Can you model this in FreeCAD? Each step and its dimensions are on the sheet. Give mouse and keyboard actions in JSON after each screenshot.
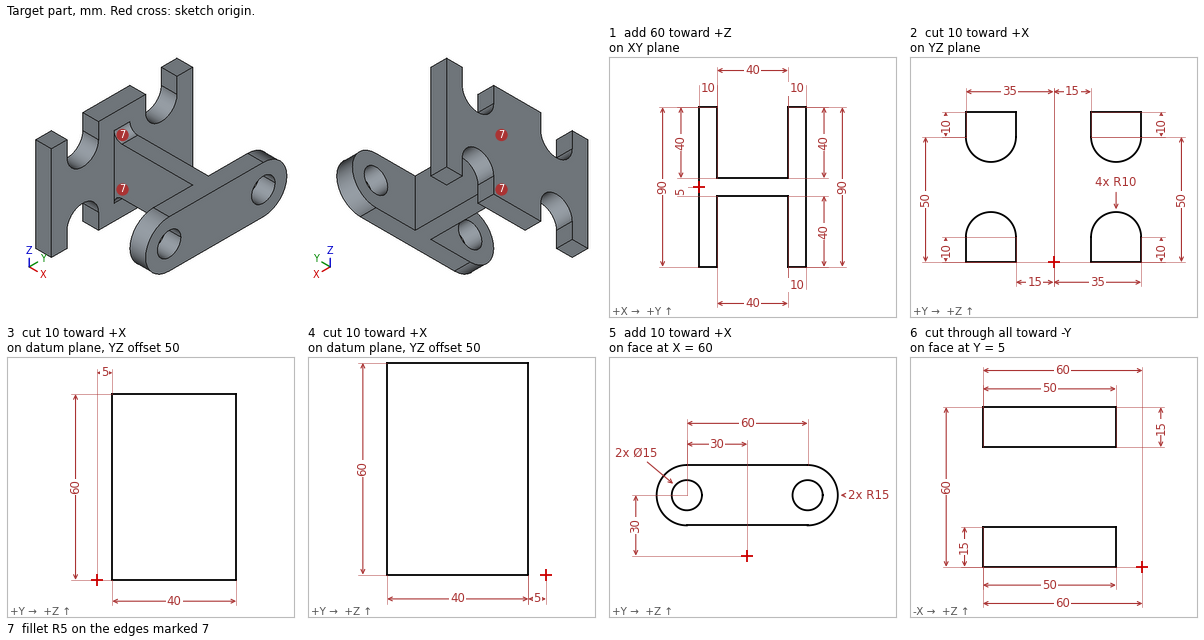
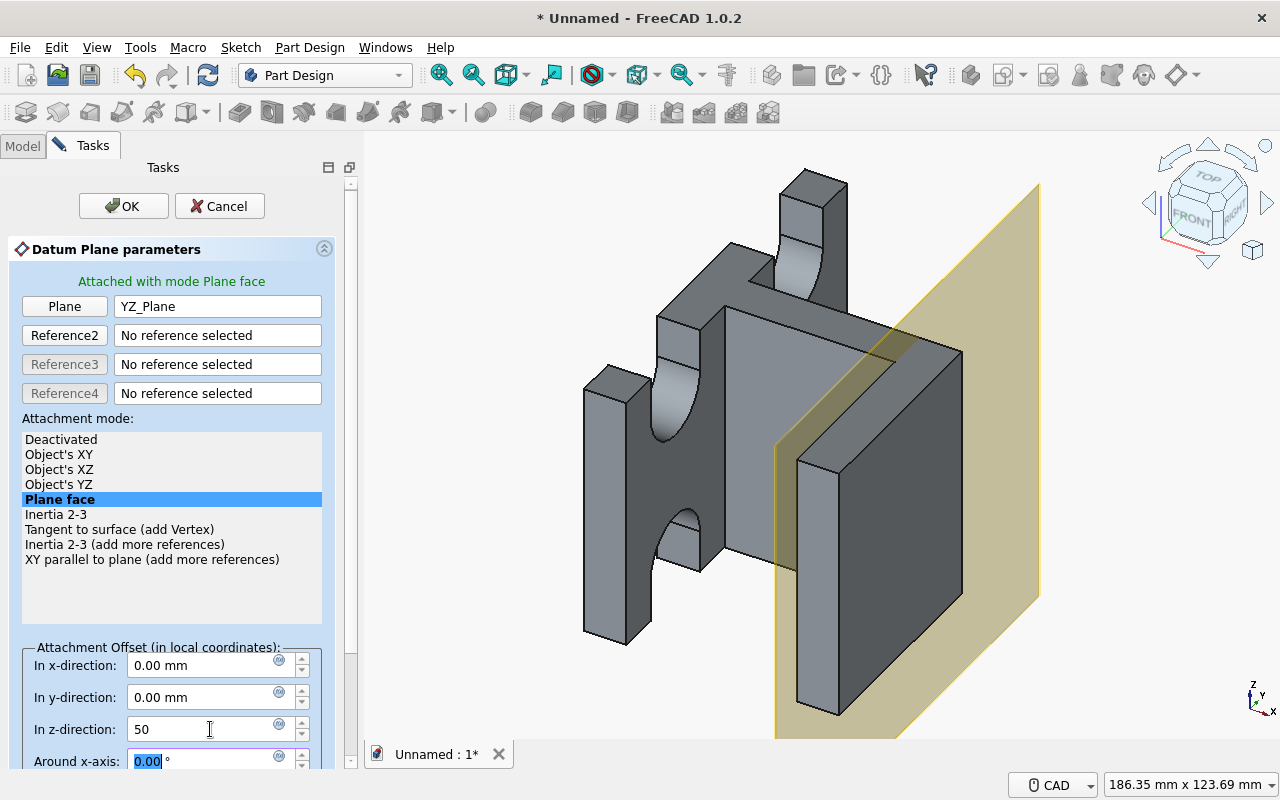
{"action": "left_click", "coordinate": [124, 206]}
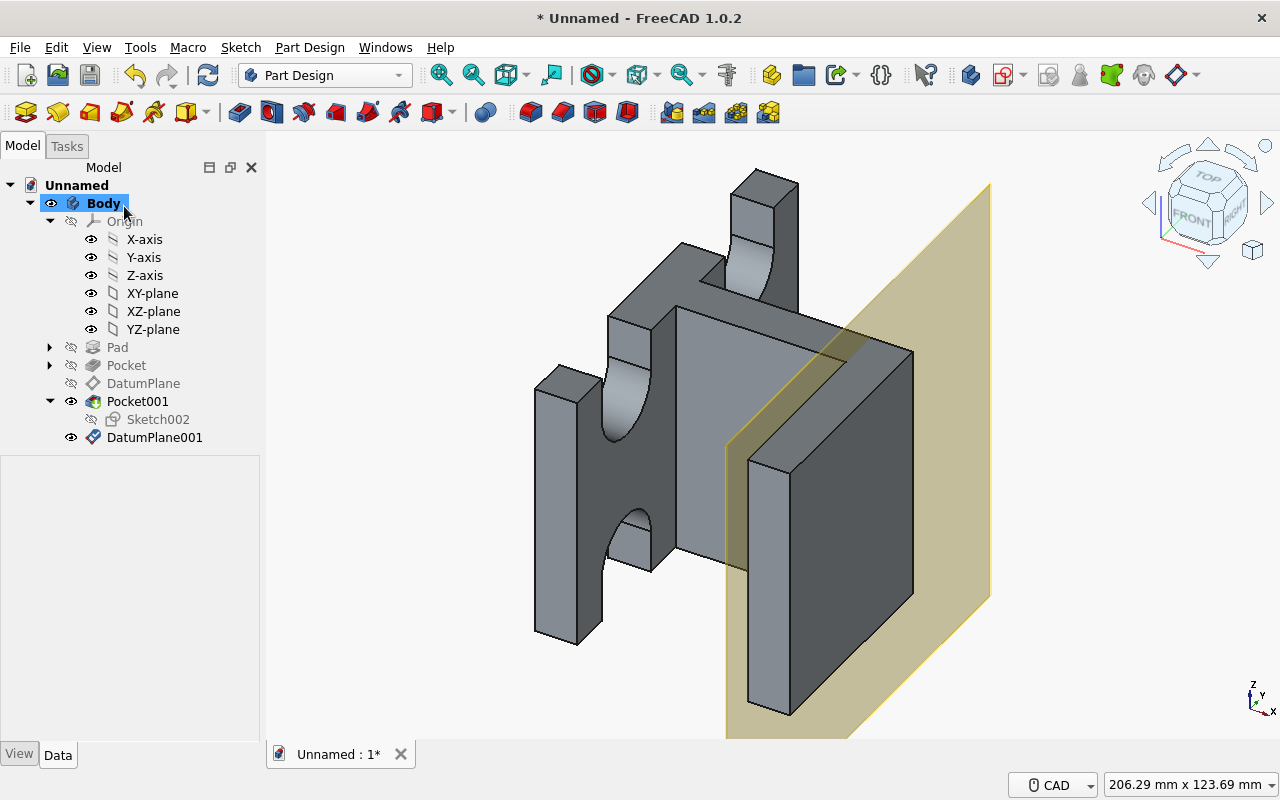
{"action": "left_click", "coordinate": [116, 437]}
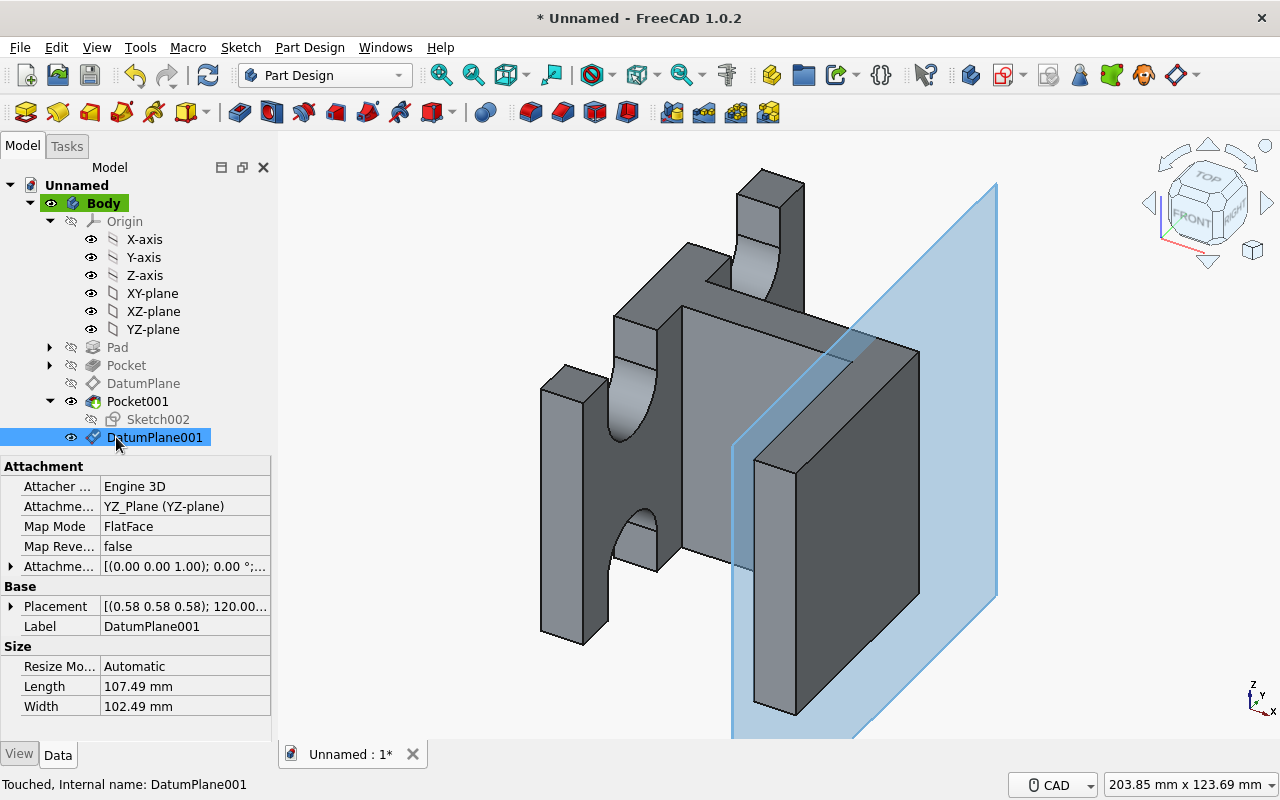
{"action": "left_click", "coordinate": [1004, 76]}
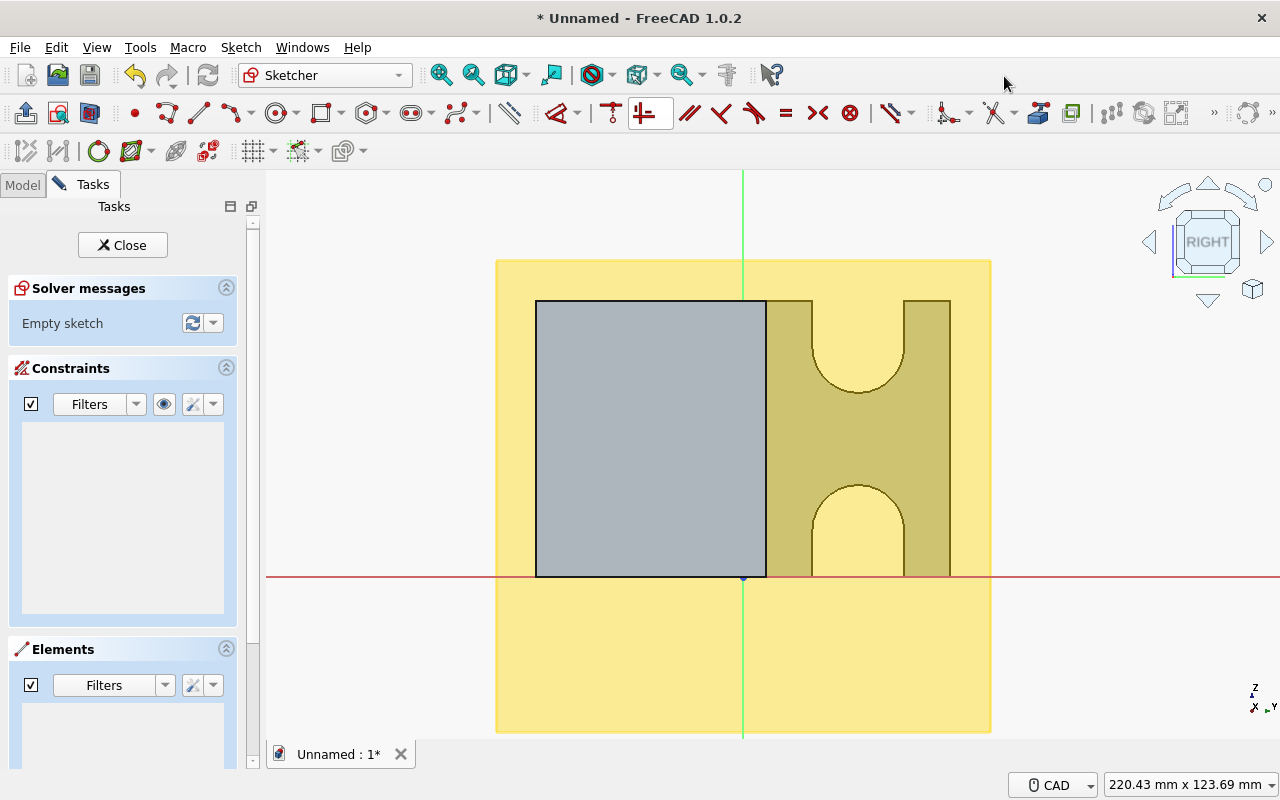
{"action": "left_click", "coordinate": [90, 114]}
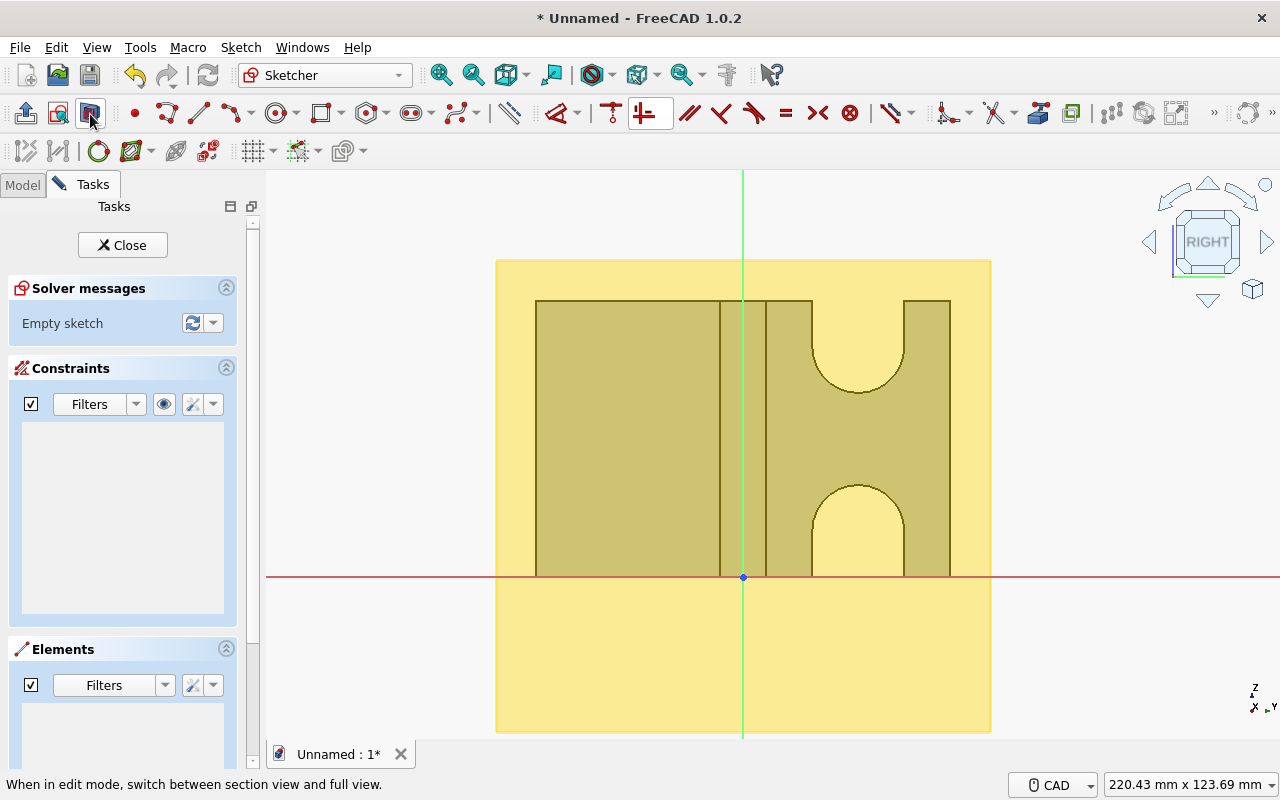
{"action": "left_click", "coordinate": [322, 114]}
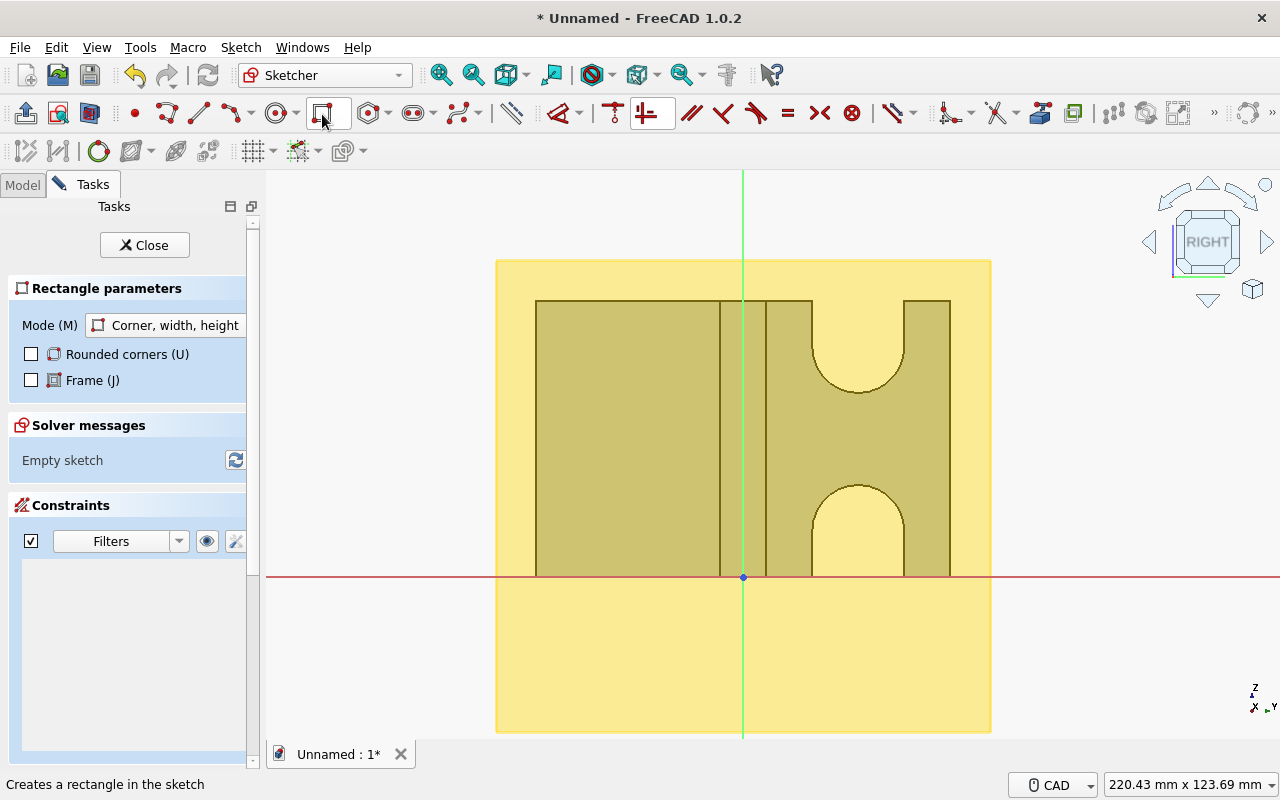
{"action": "left_click", "coordinate": [536, 301]}
{"action": "left_click", "coordinate": [720, 577]}
{"action": "key", "text": "Escape"}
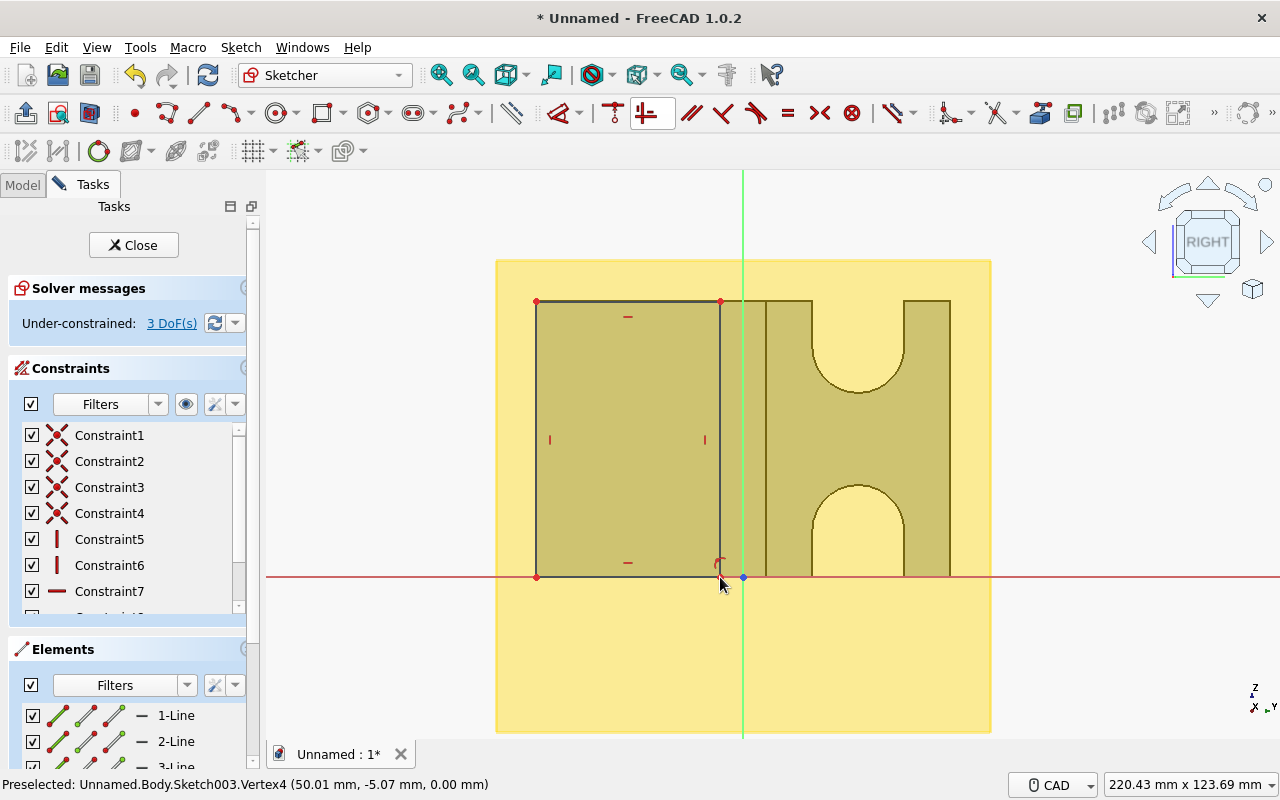
{"action": "left_click", "coordinate": [558, 114]}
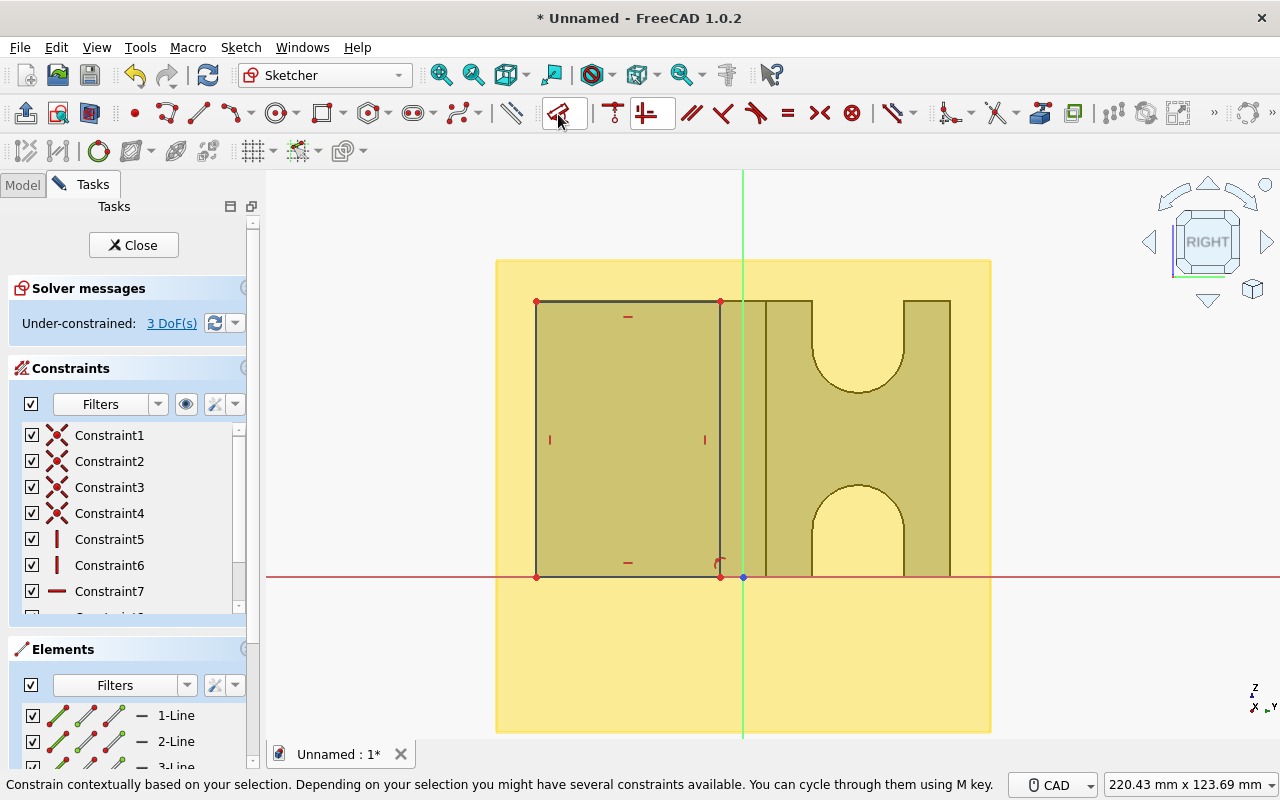
{"action": "left_click", "coordinate": [536, 385]}
{"action": "left_click", "coordinate": [502, 440]}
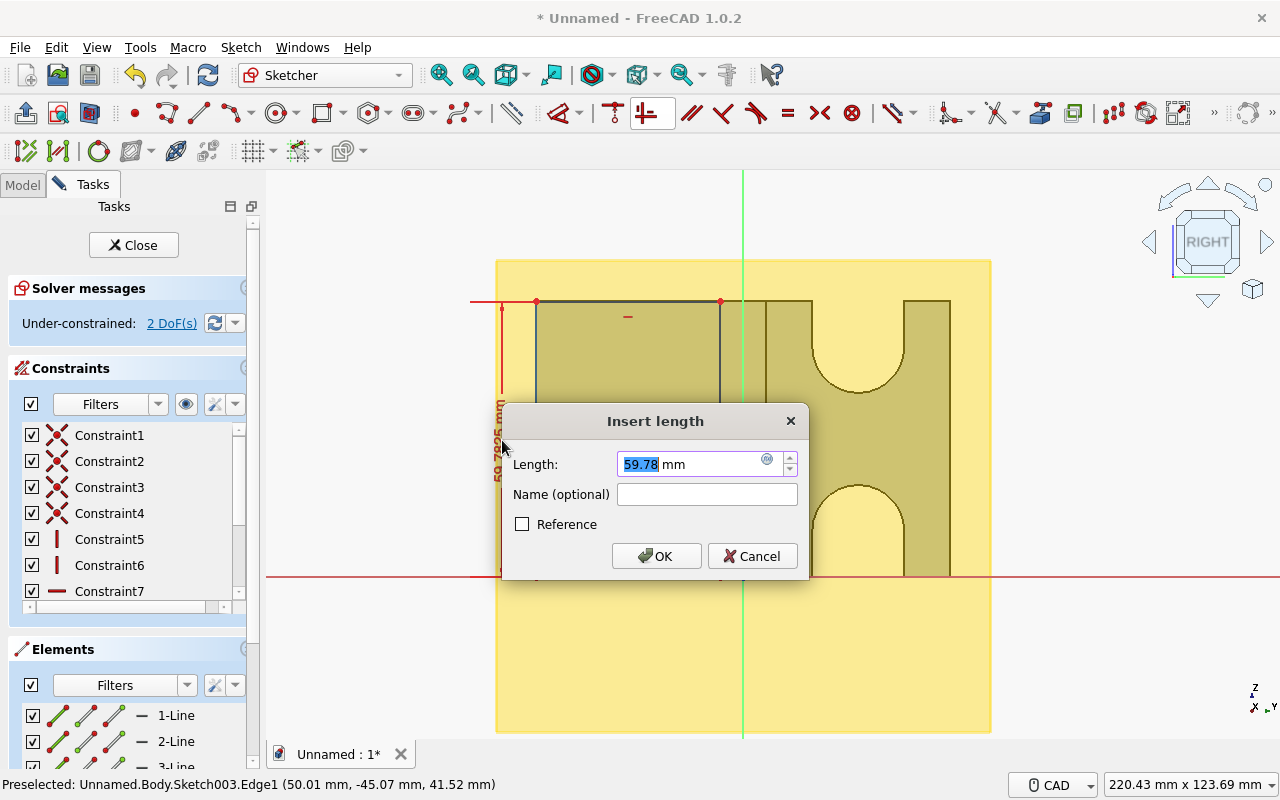
{"action": "type", "text": "60"}
{"action": "key", "text": "Return"}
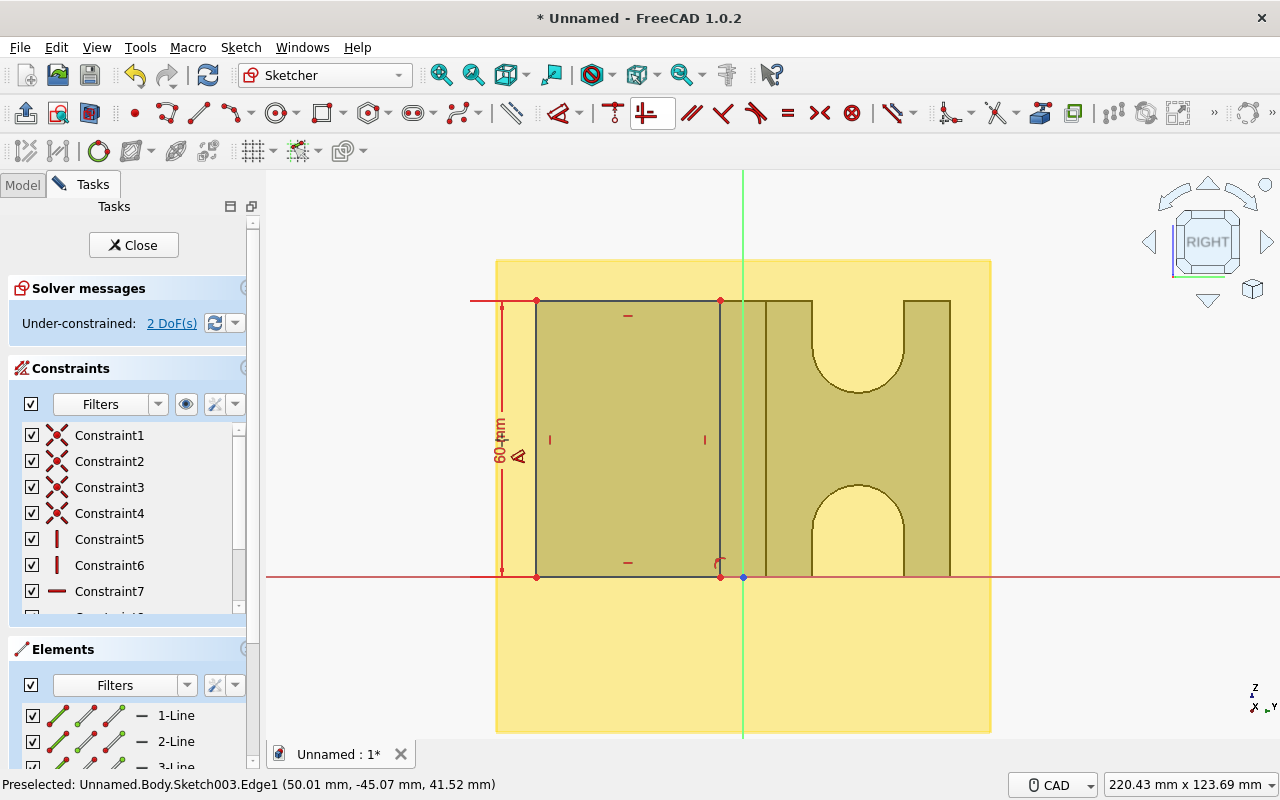
{"action": "left_click", "coordinate": [591, 577]}
{"action": "left_click", "coordinate": [628, 611]}